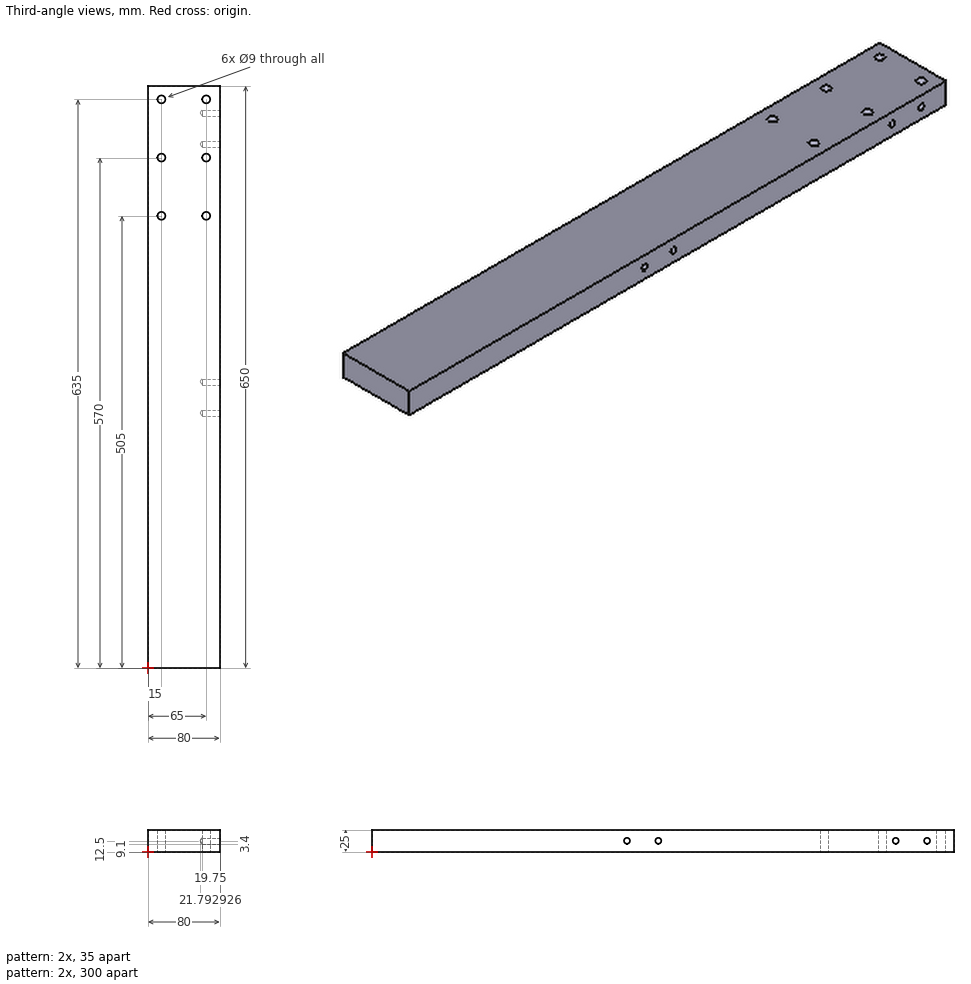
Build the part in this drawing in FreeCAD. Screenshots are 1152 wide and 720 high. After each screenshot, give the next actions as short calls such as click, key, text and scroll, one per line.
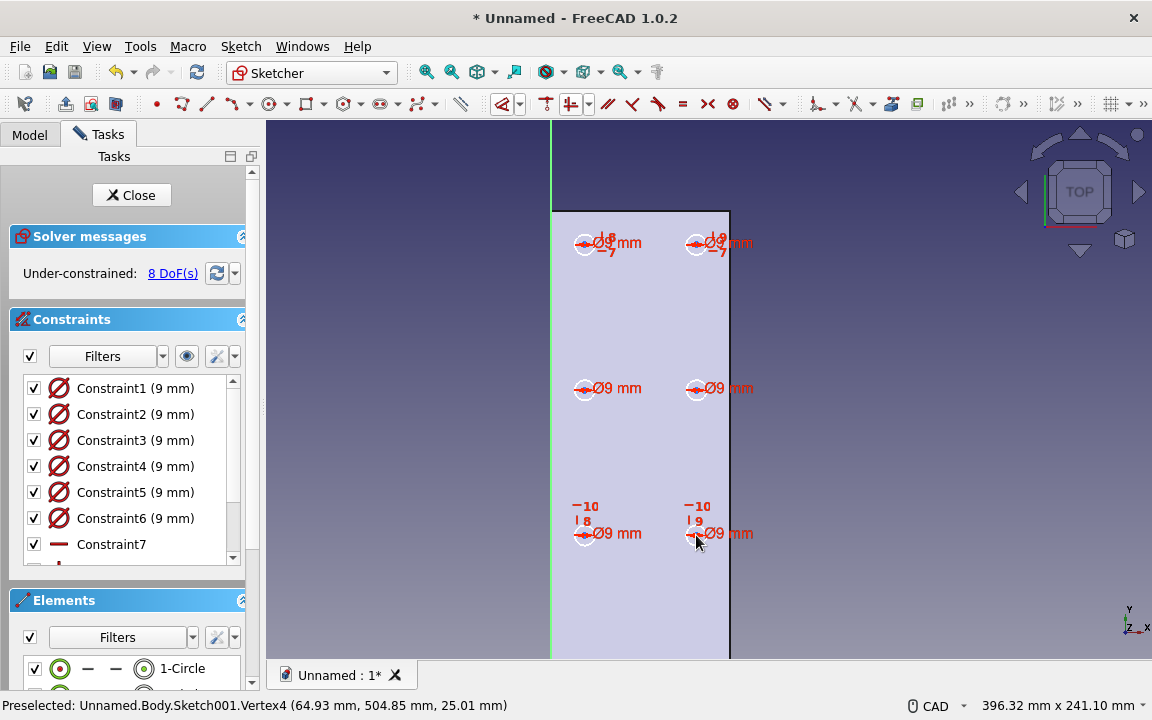
click(585, 245)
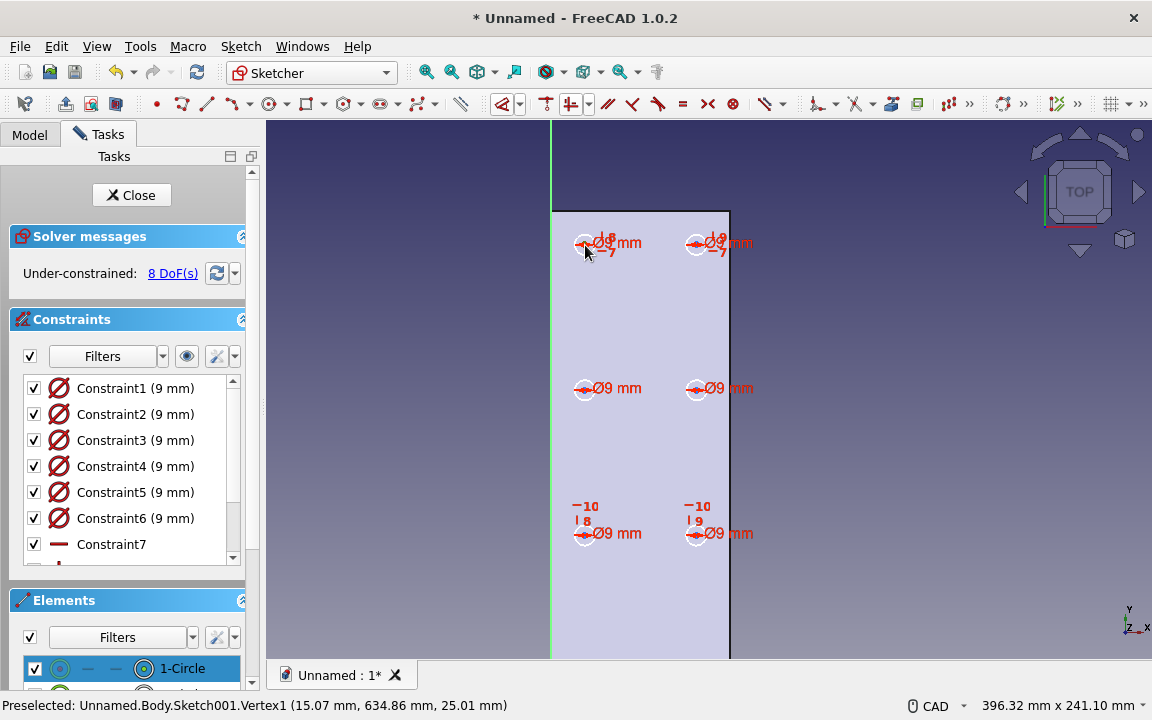
click(585, 390)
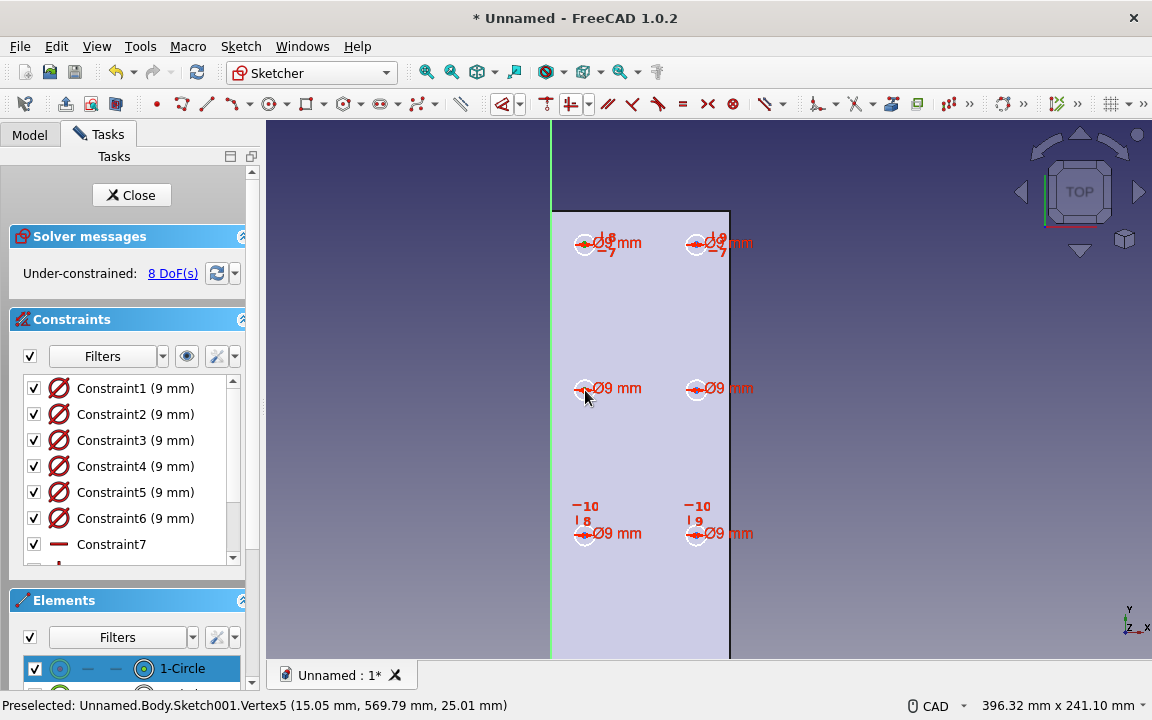
key(v)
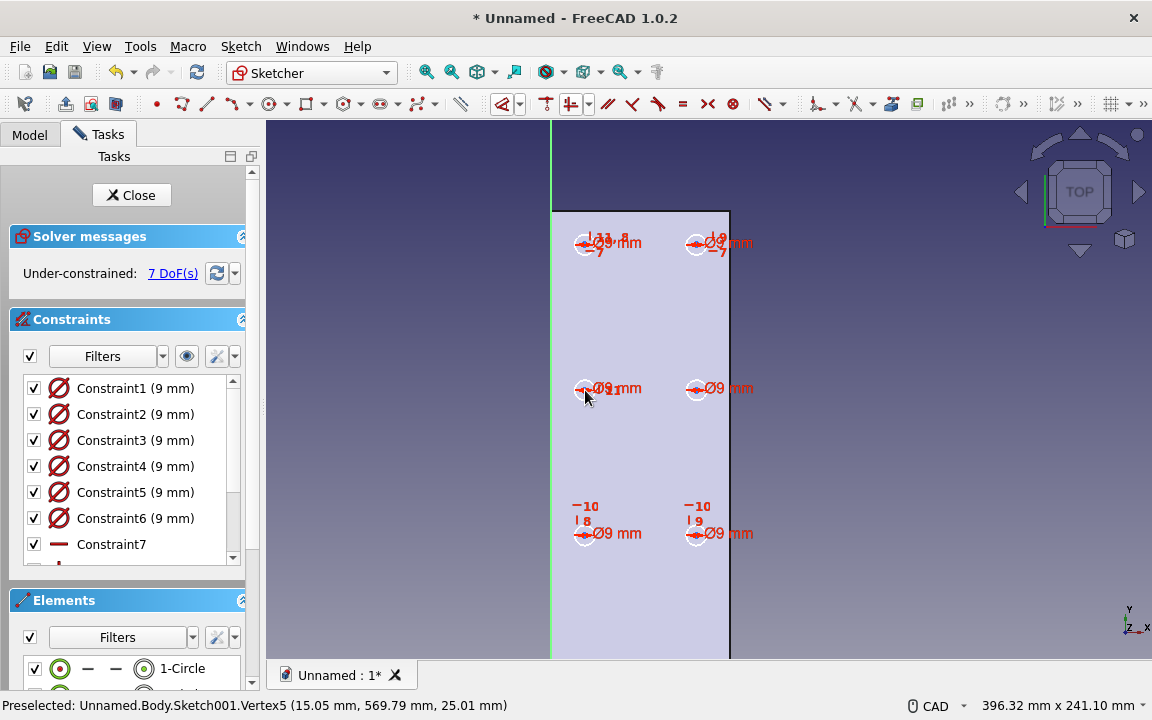
click(696, 245)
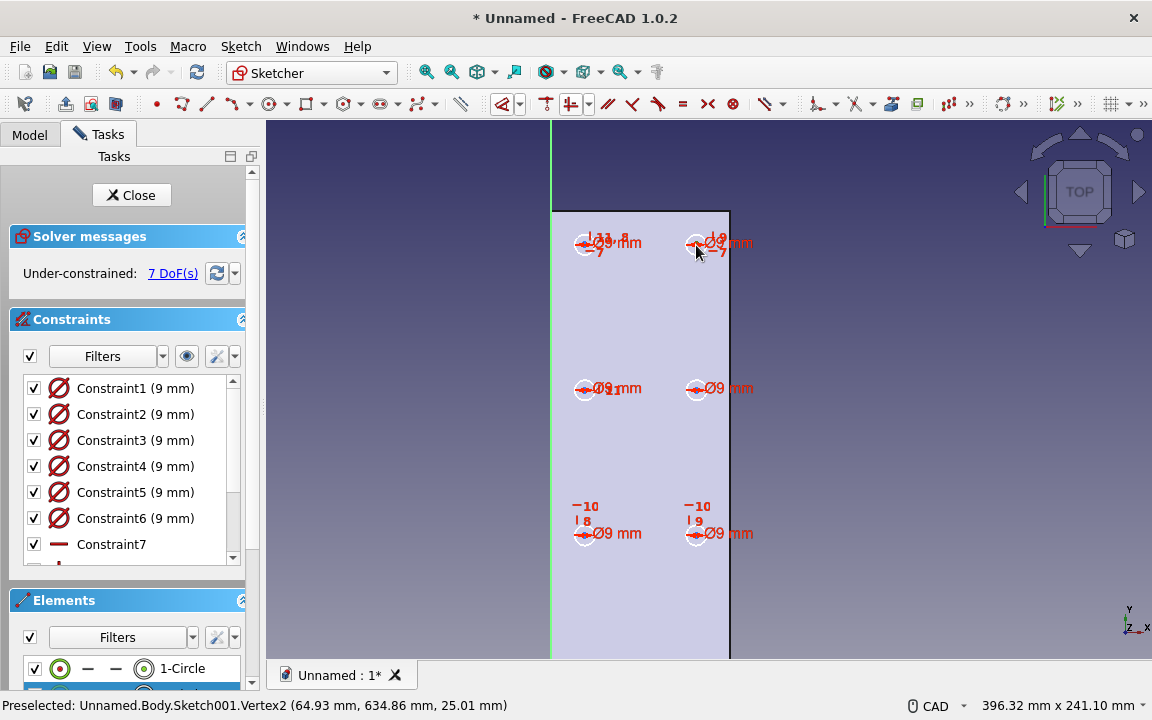
click(697, 390)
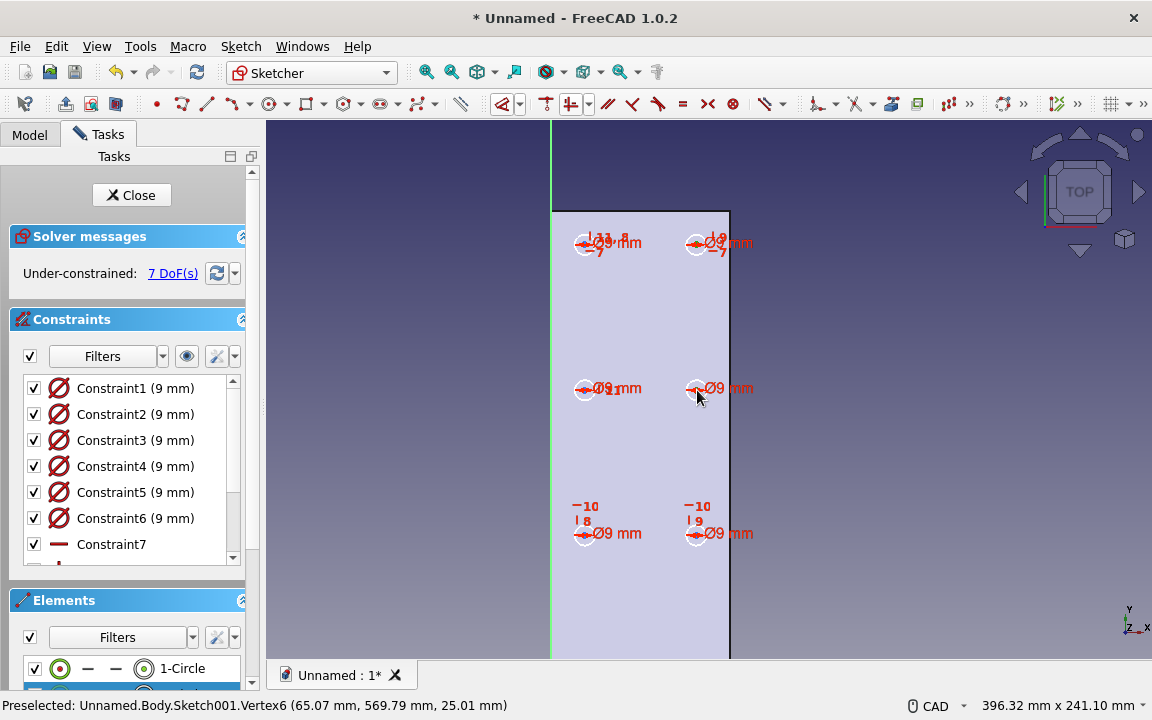
key(v)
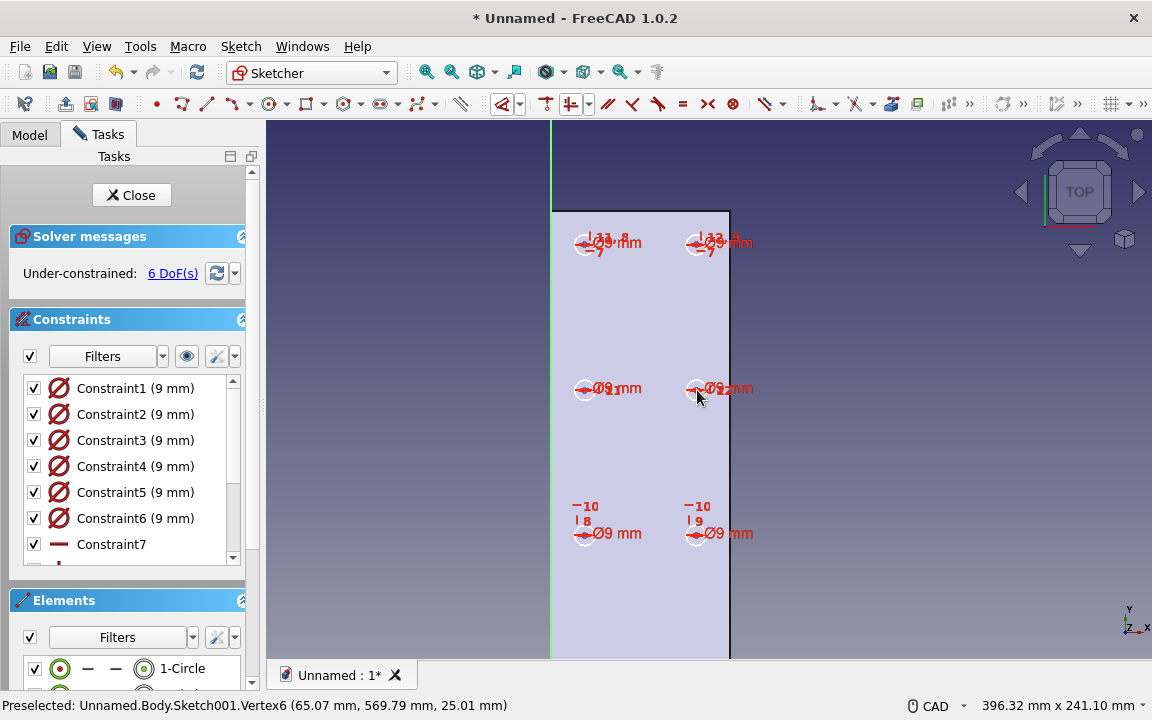
click(585, 390)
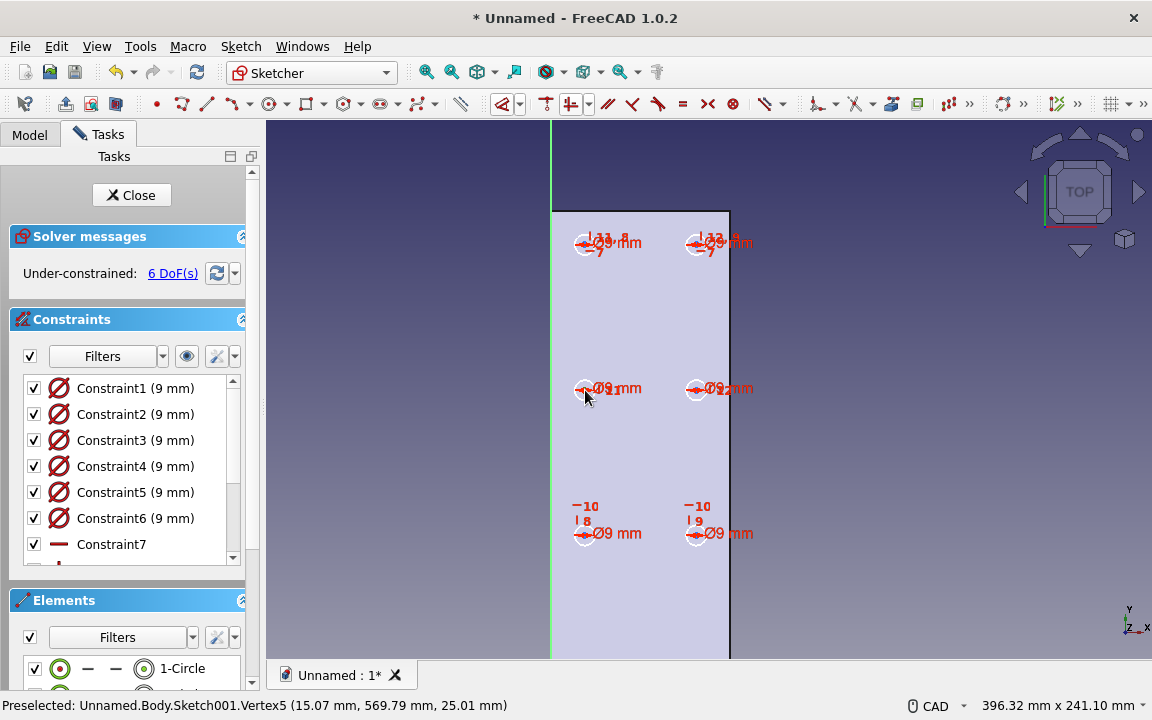
click(696, 390)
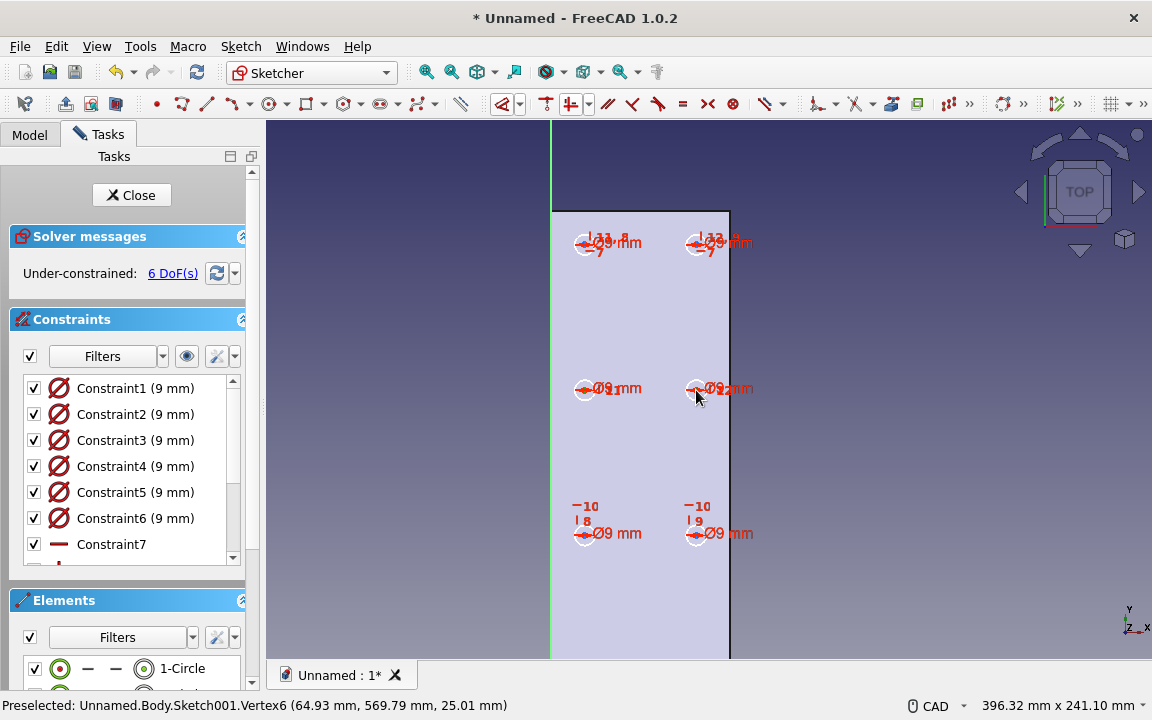
key(h)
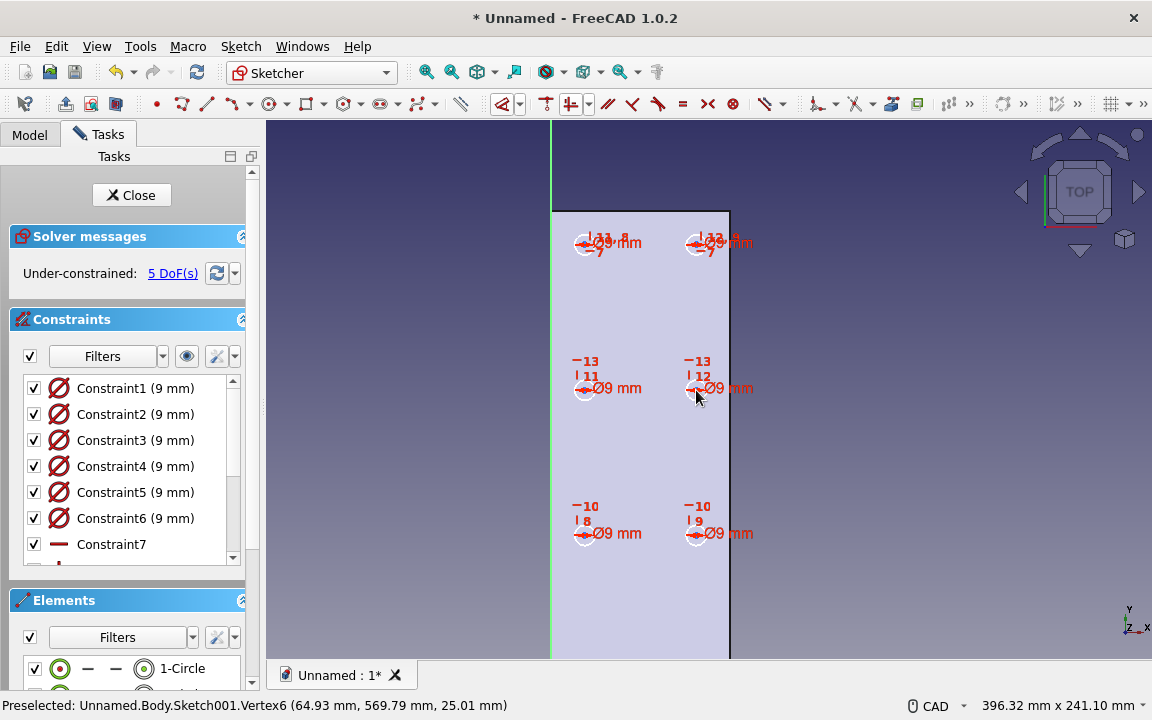
key(d)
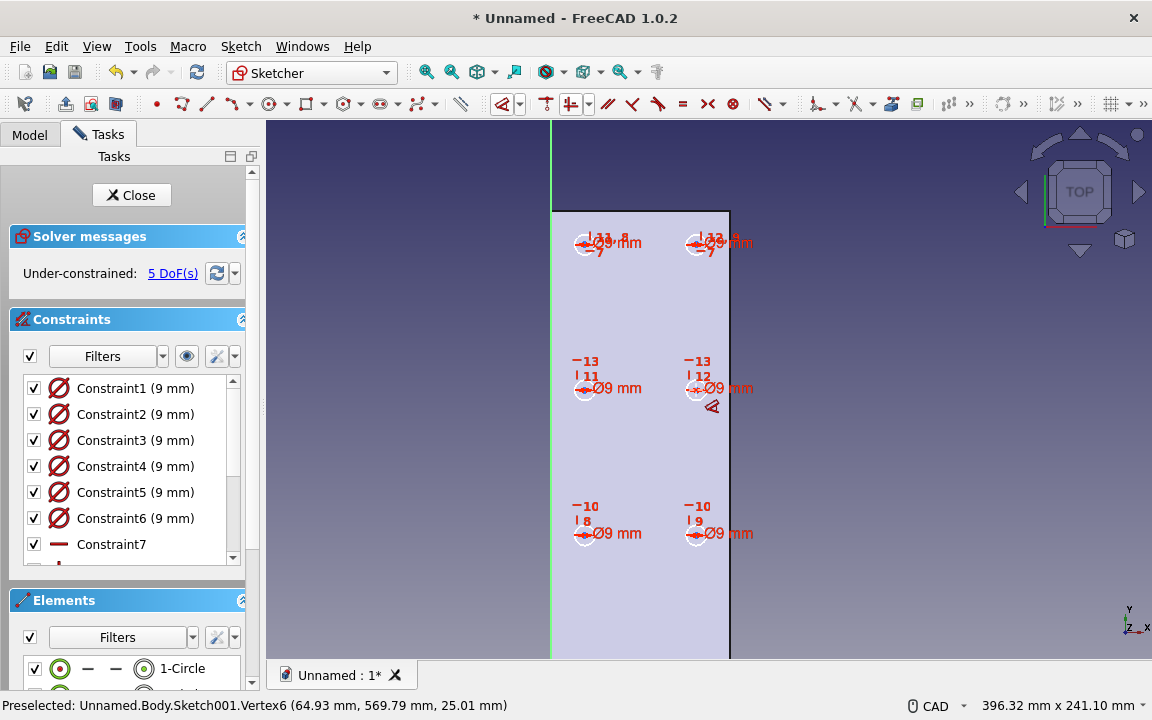
click(585, 245)
click(568, 211)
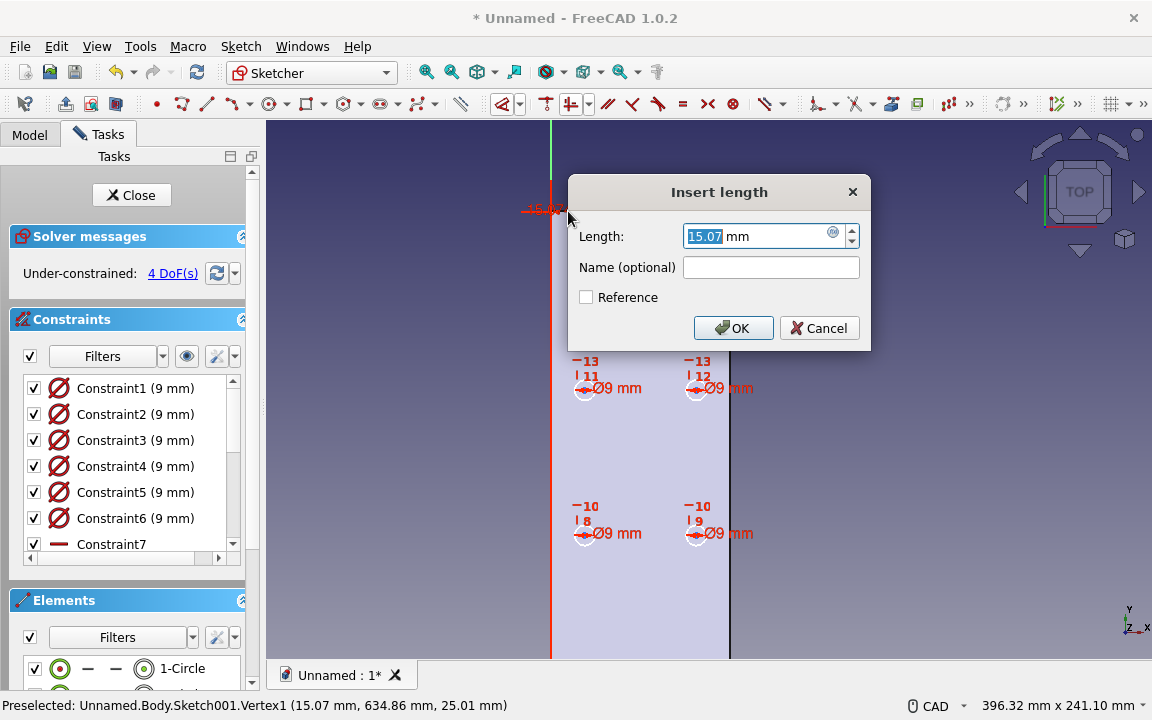
text(15)
key(Return)